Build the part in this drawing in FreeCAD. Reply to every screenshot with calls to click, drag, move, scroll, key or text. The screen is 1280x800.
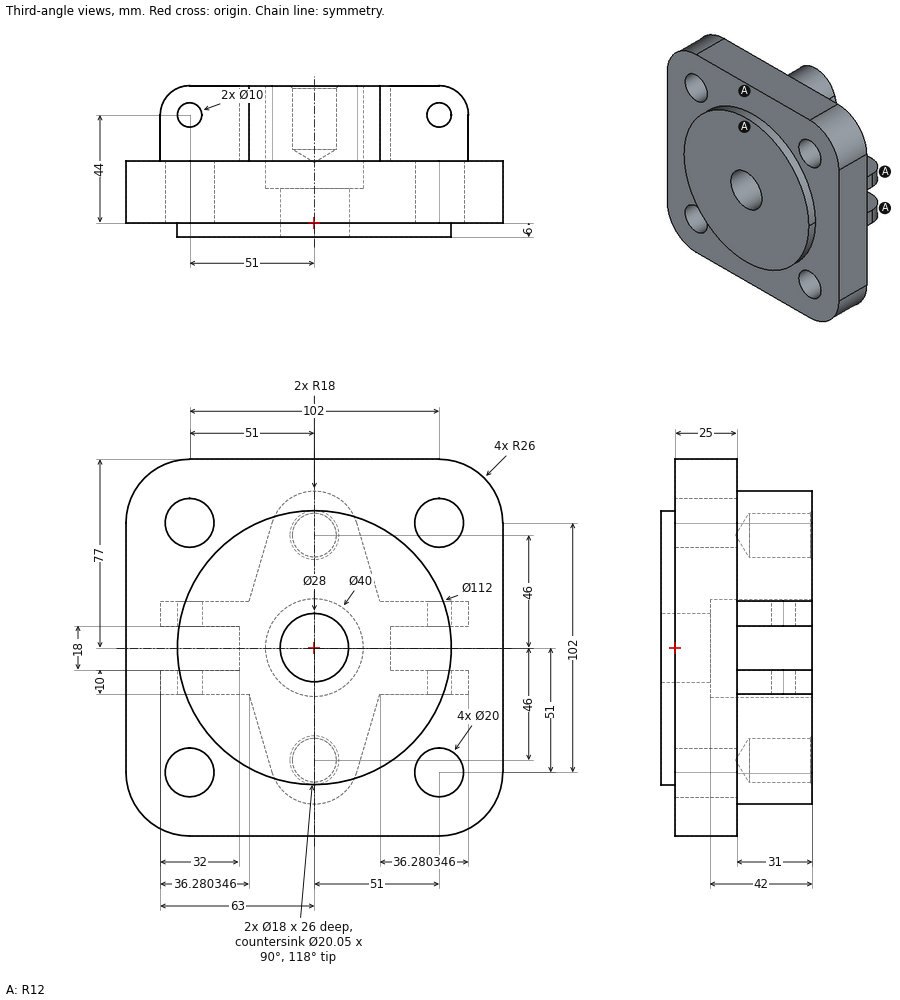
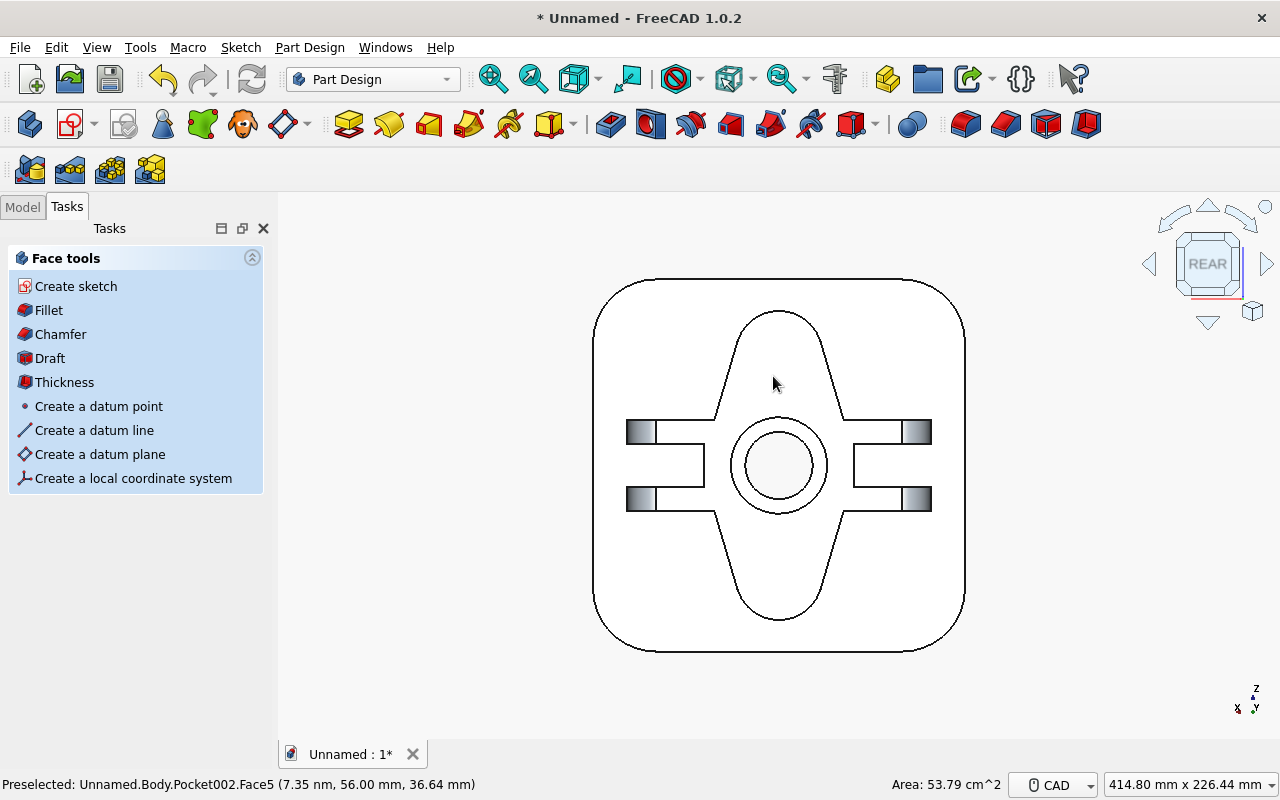
click(70, 124)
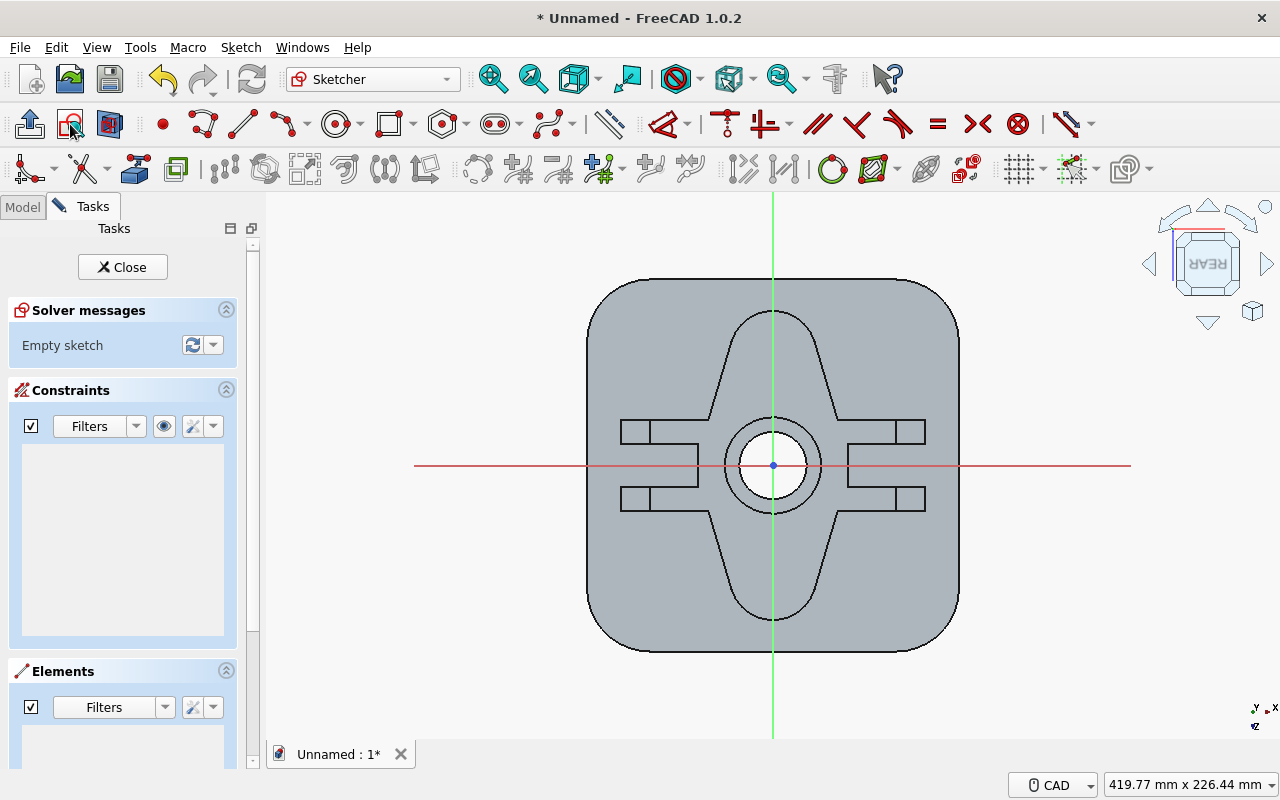
key(g)
key(c)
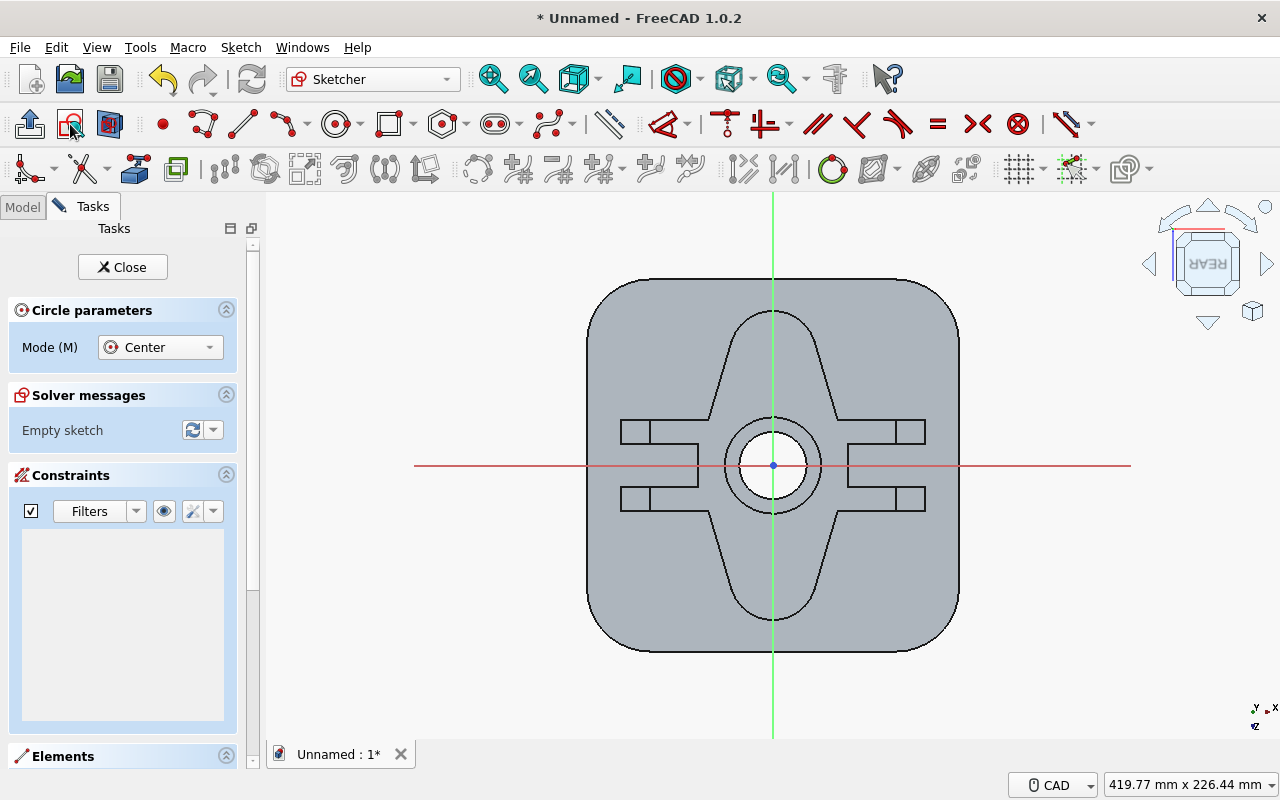
click(773, 354)
click(788, 339)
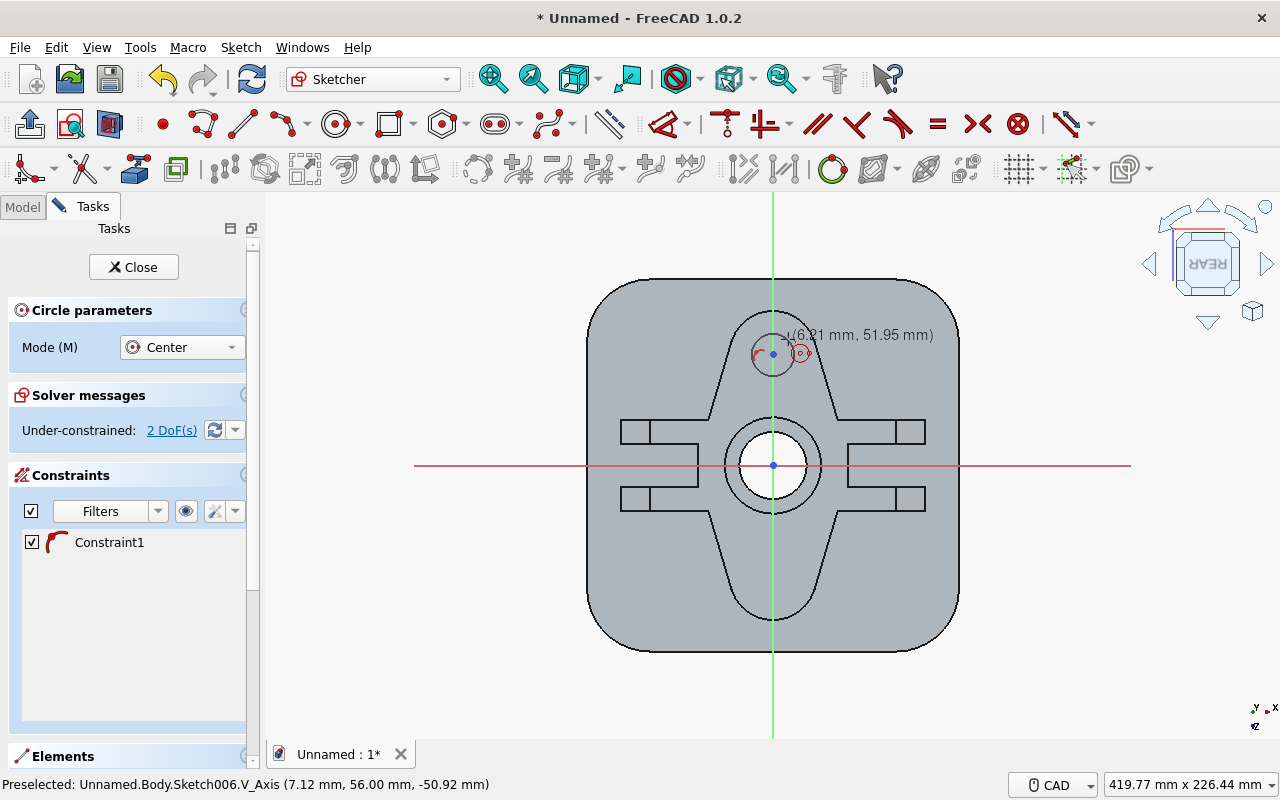
click(773, 577)
click(788, 561)
key(Escape)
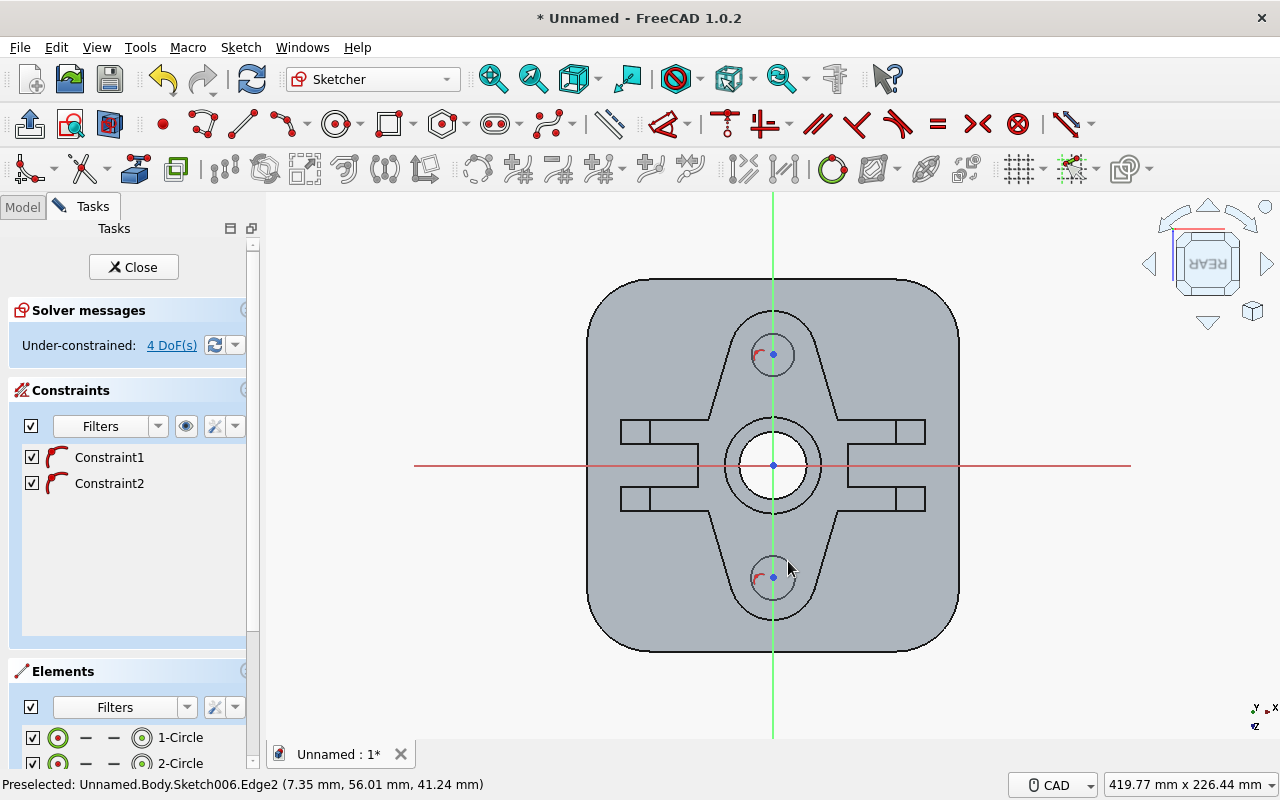
click(788, 340)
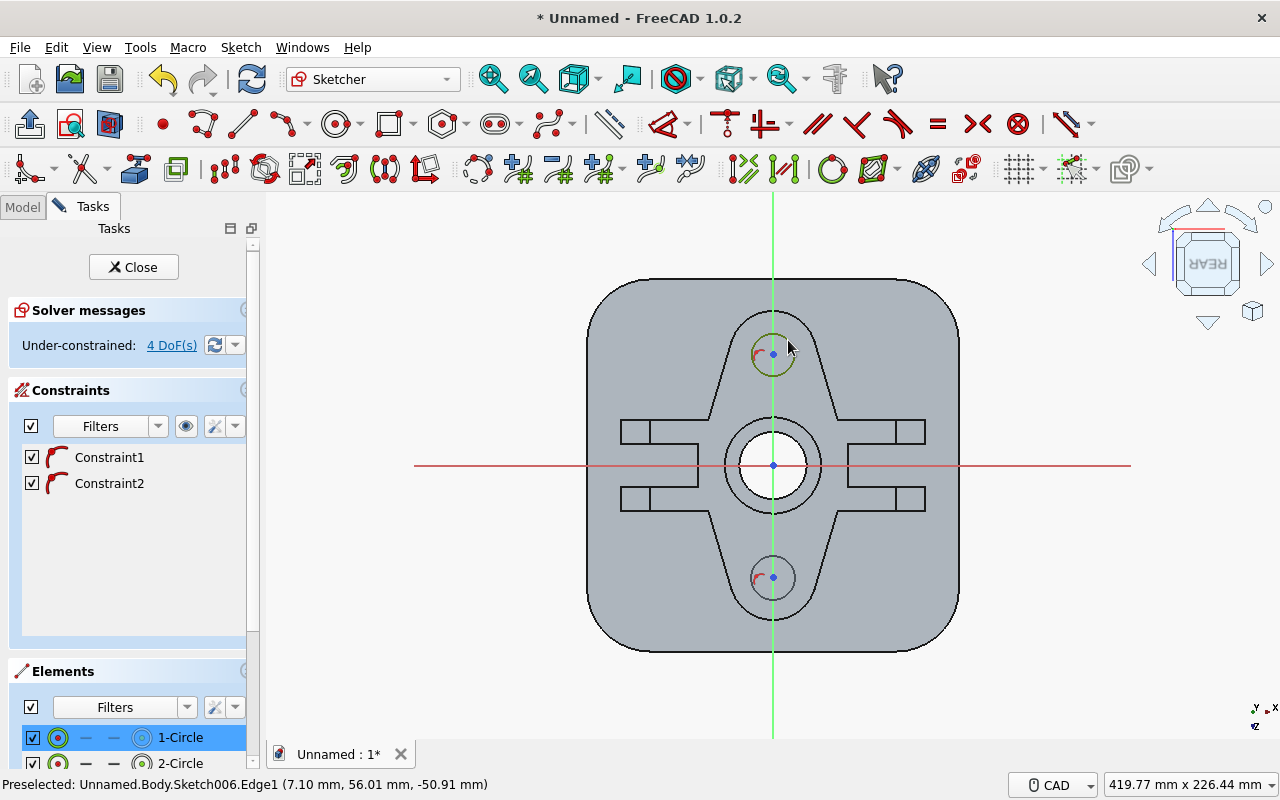
click(788, 562)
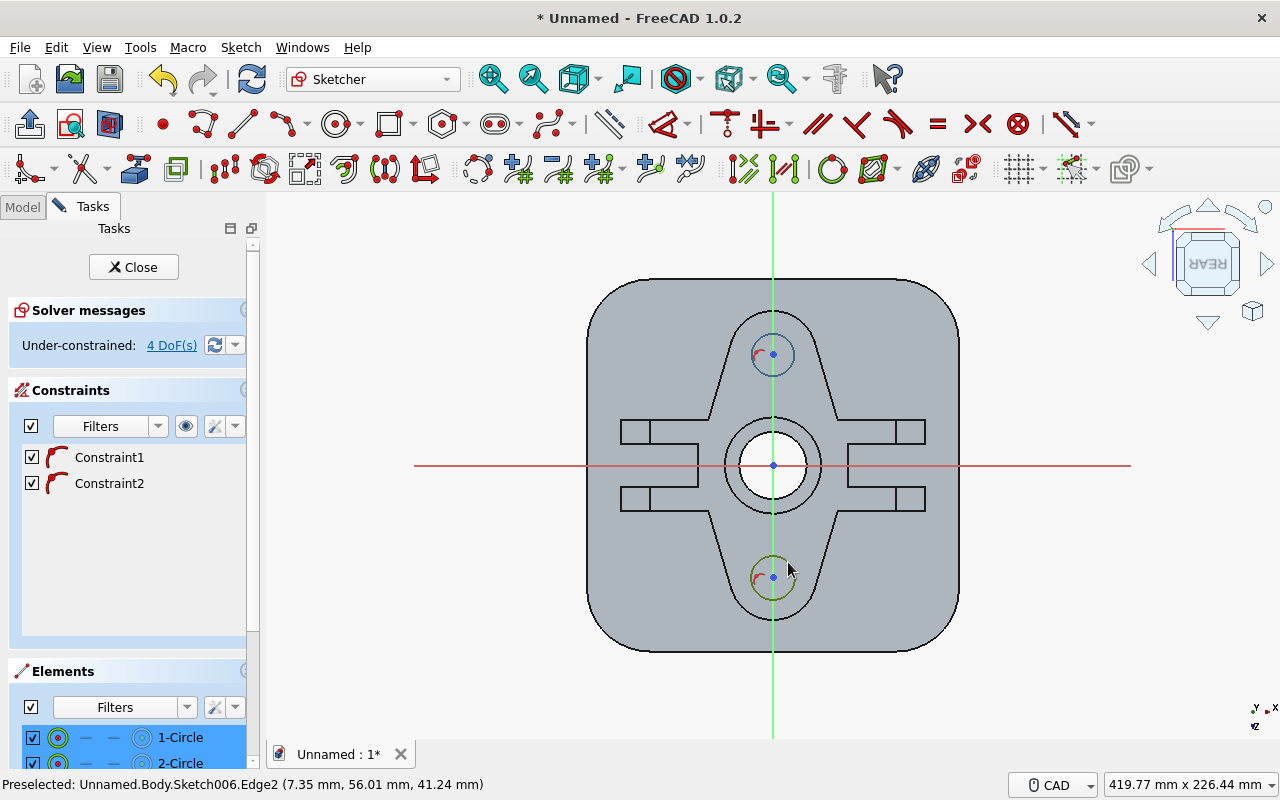
key(e)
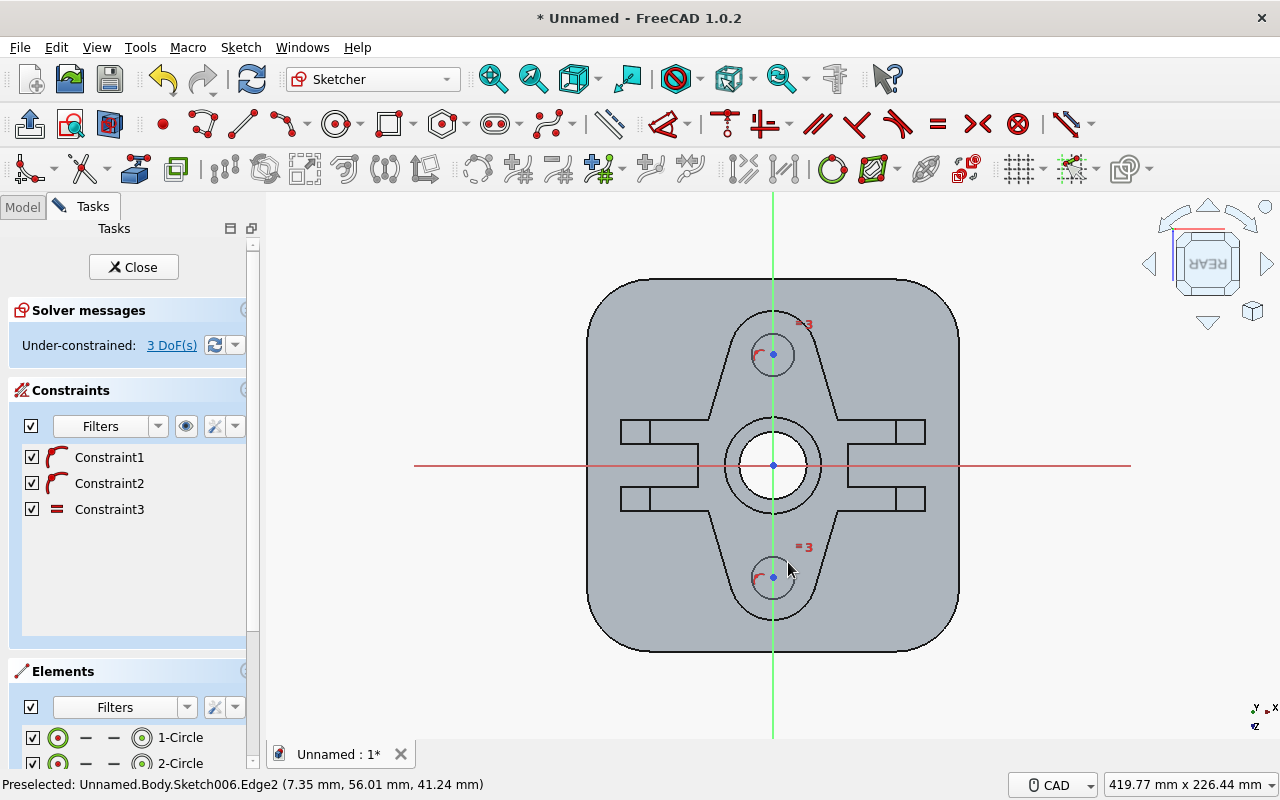
key(d)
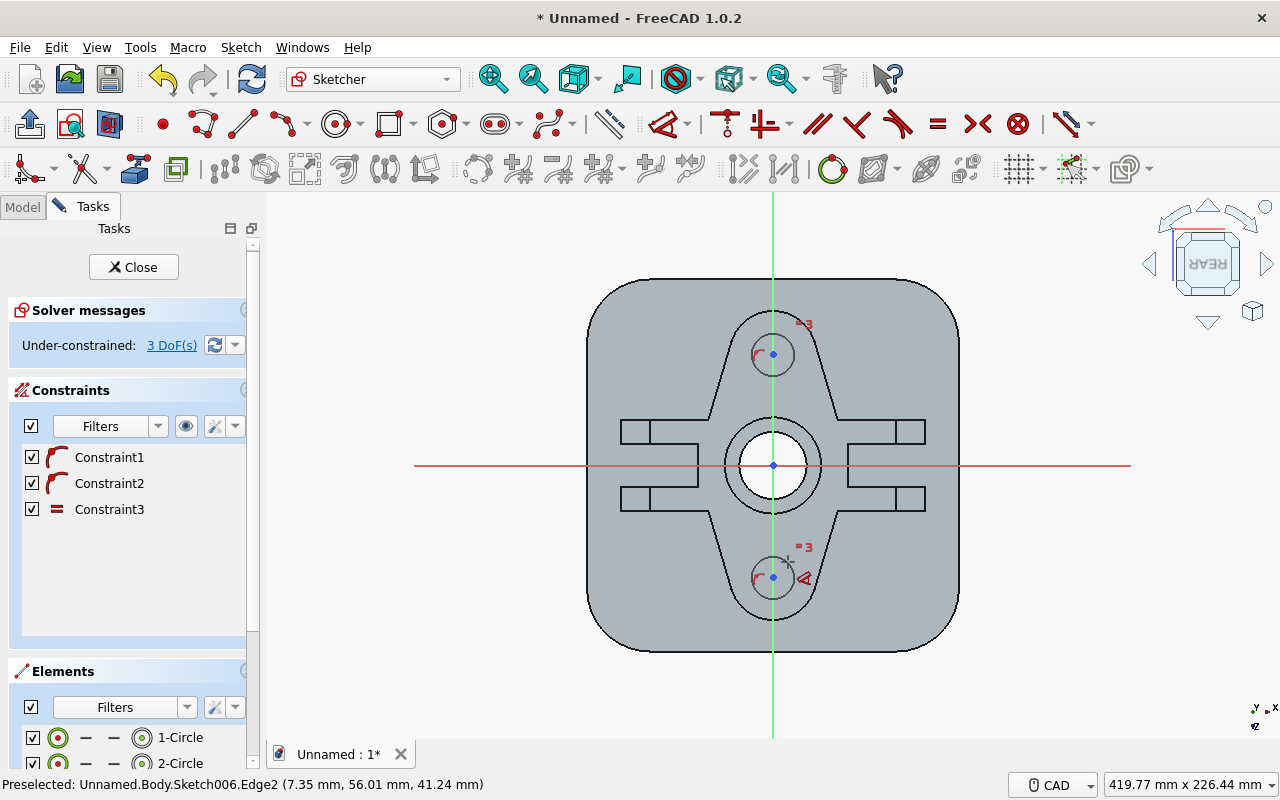
click(788, 340)
click(811, 317)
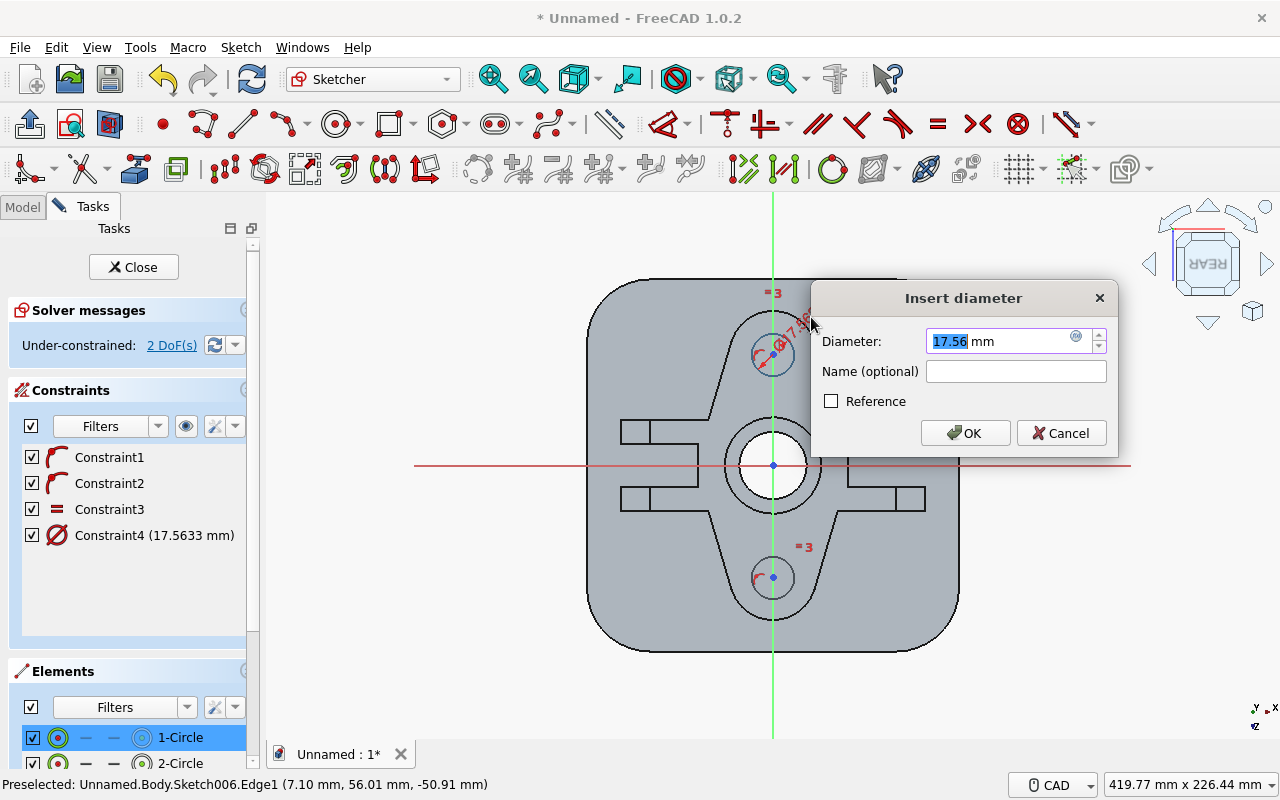
text(18)
key(Return)